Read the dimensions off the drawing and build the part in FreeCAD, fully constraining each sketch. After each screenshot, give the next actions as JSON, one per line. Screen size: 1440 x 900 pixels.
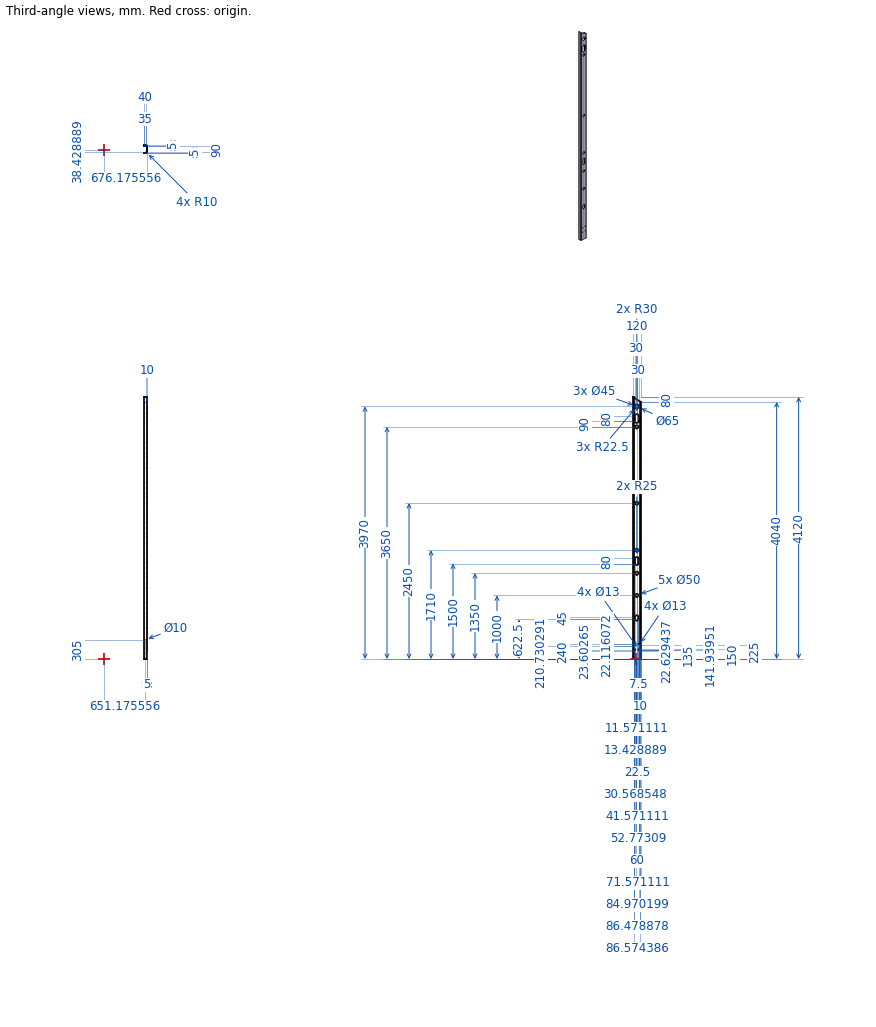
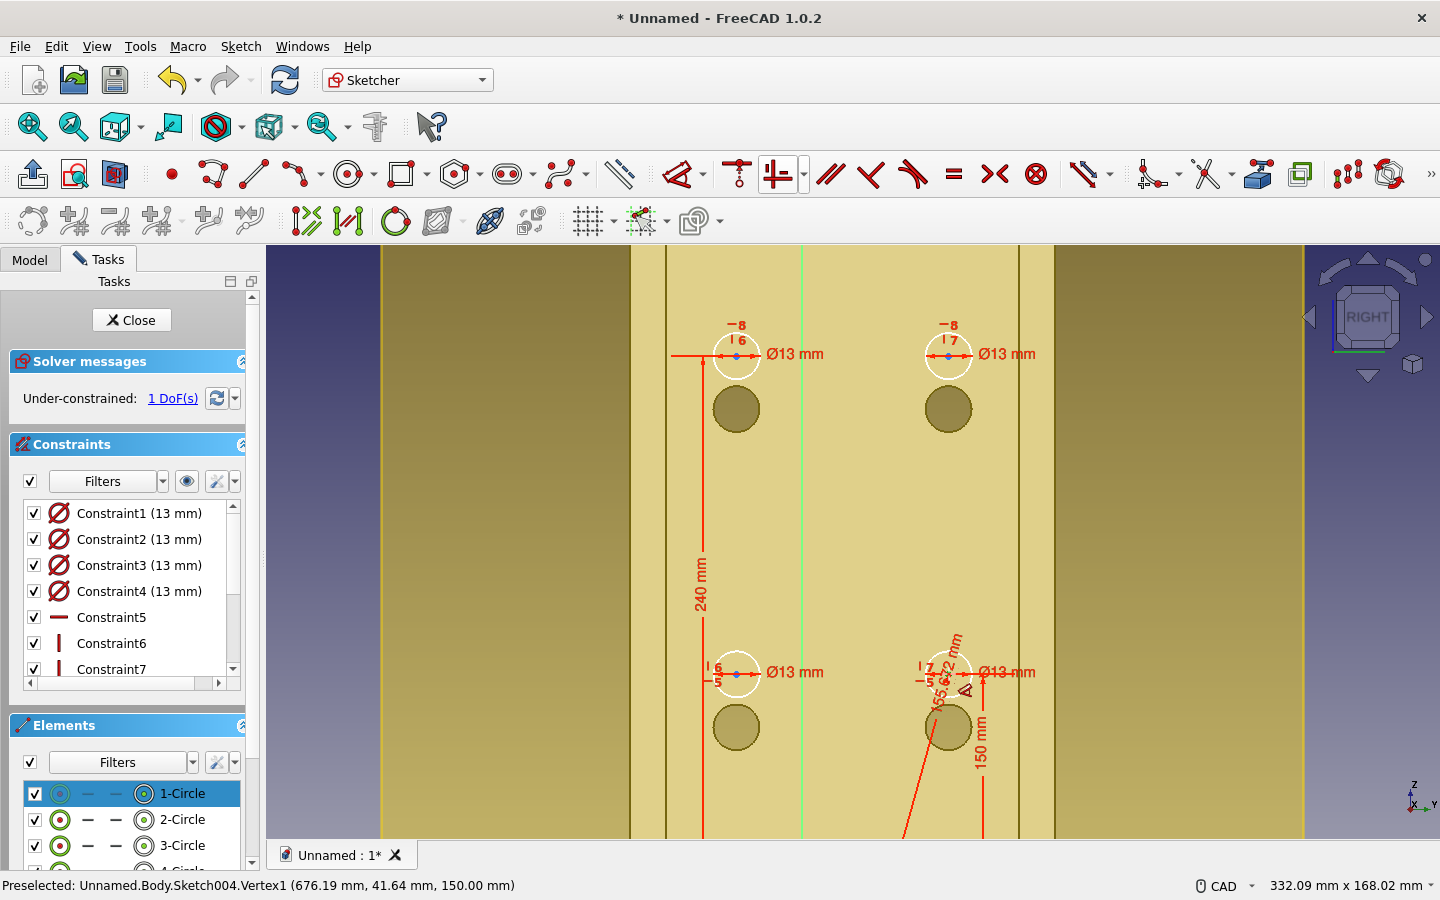
{"action": "left_click", "coordinate": [737, 674]}
{"action": "left_click", "coordinate": [843, 640]}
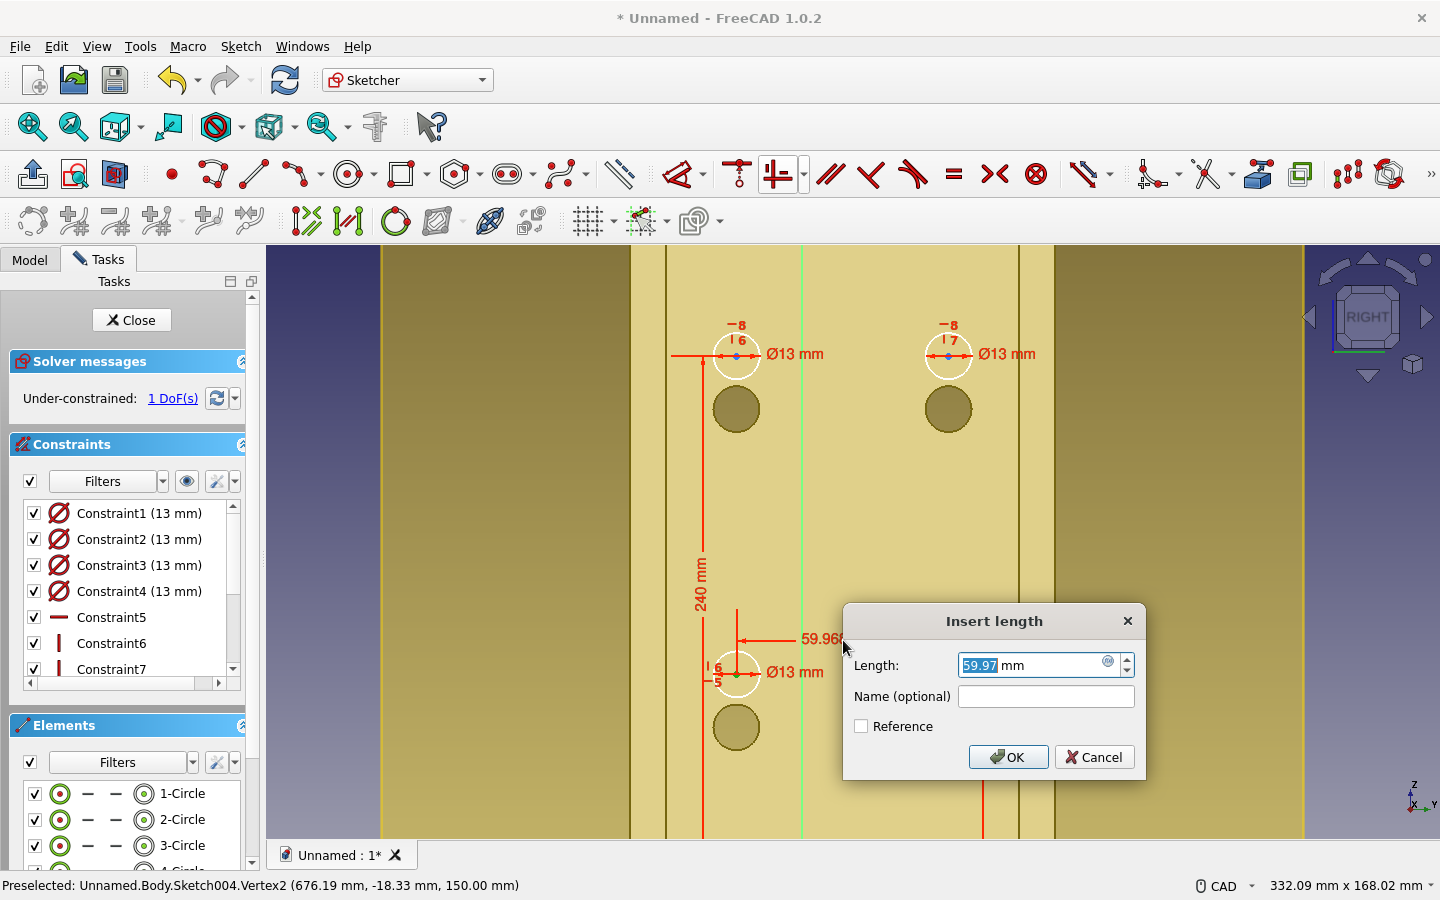
{"action": "type", "text": "60"}
{"action": "key", "text": "Return"}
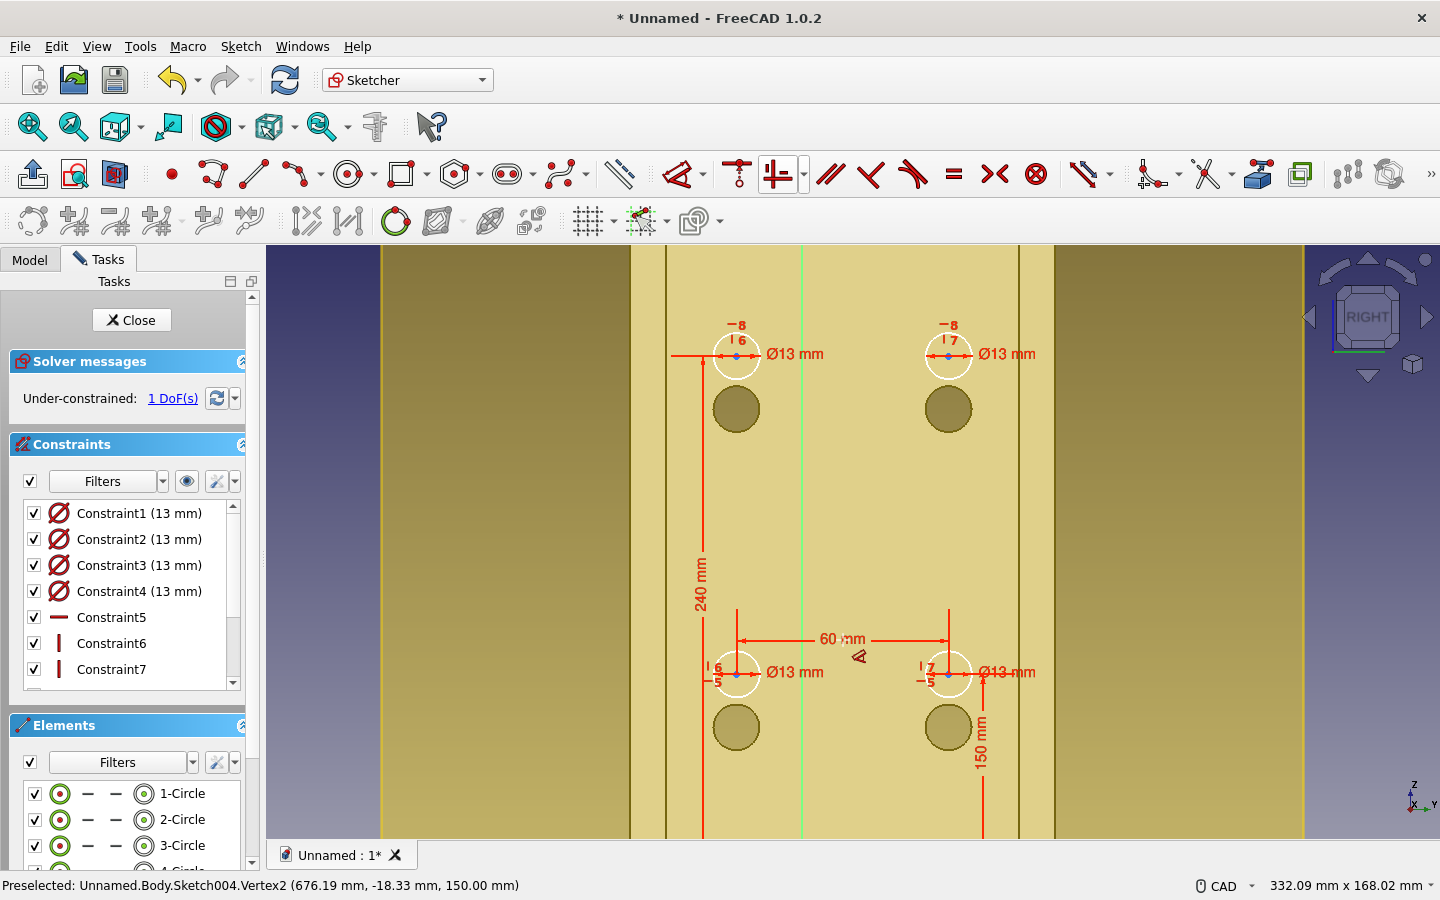
{"action": "left_click", "coordinate": [949, 674]}
{"action": "left_click", "coordinate": [927, 640]}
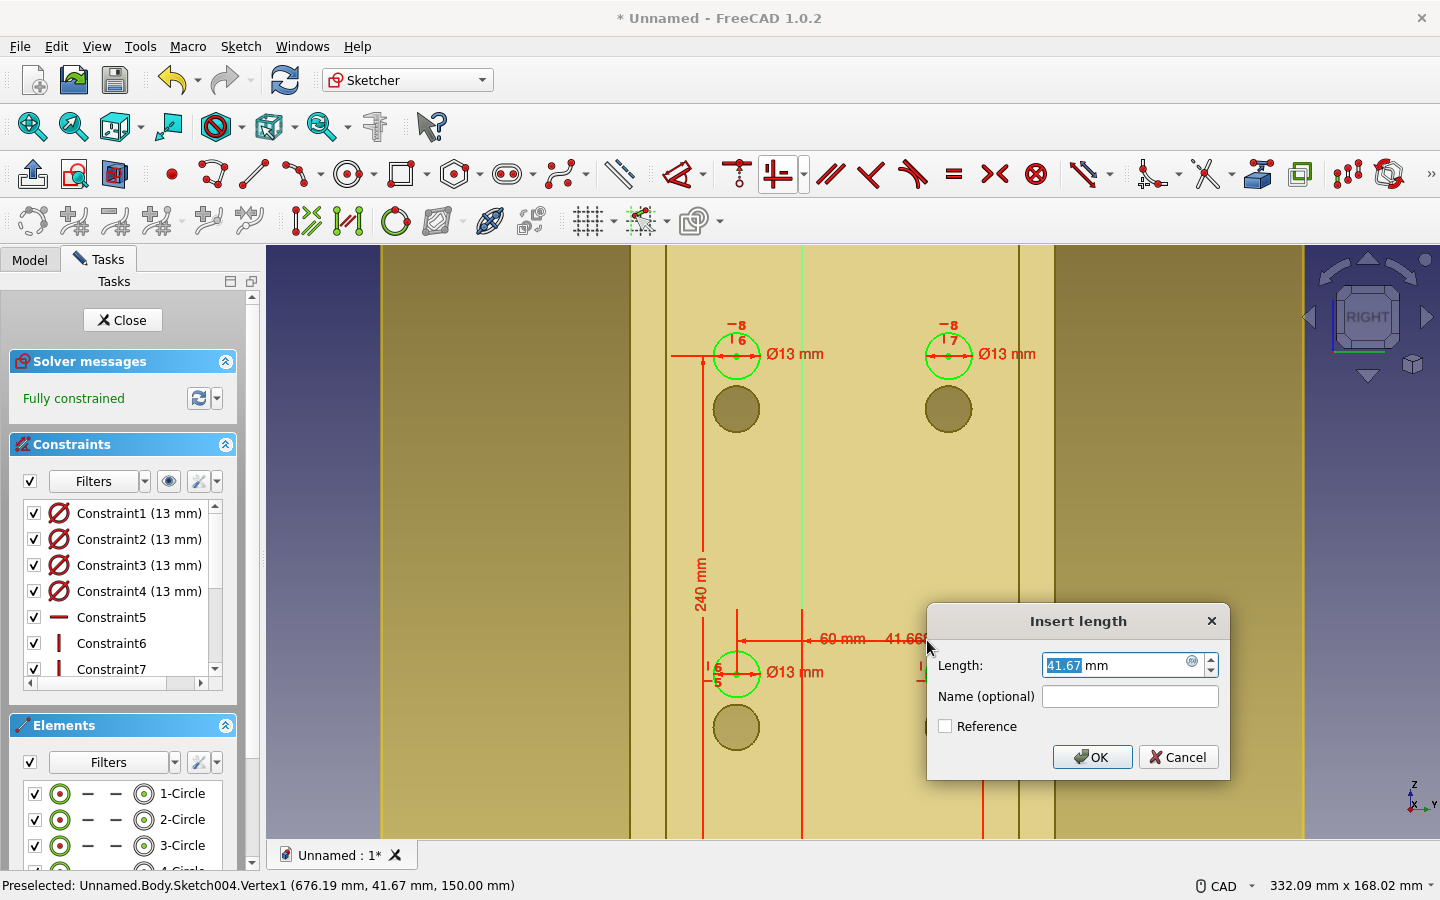
{"action": "type", "text": "41.571111"}
{"action": "key", "text": "Return"}
{"action": "key", "text": "Escape"}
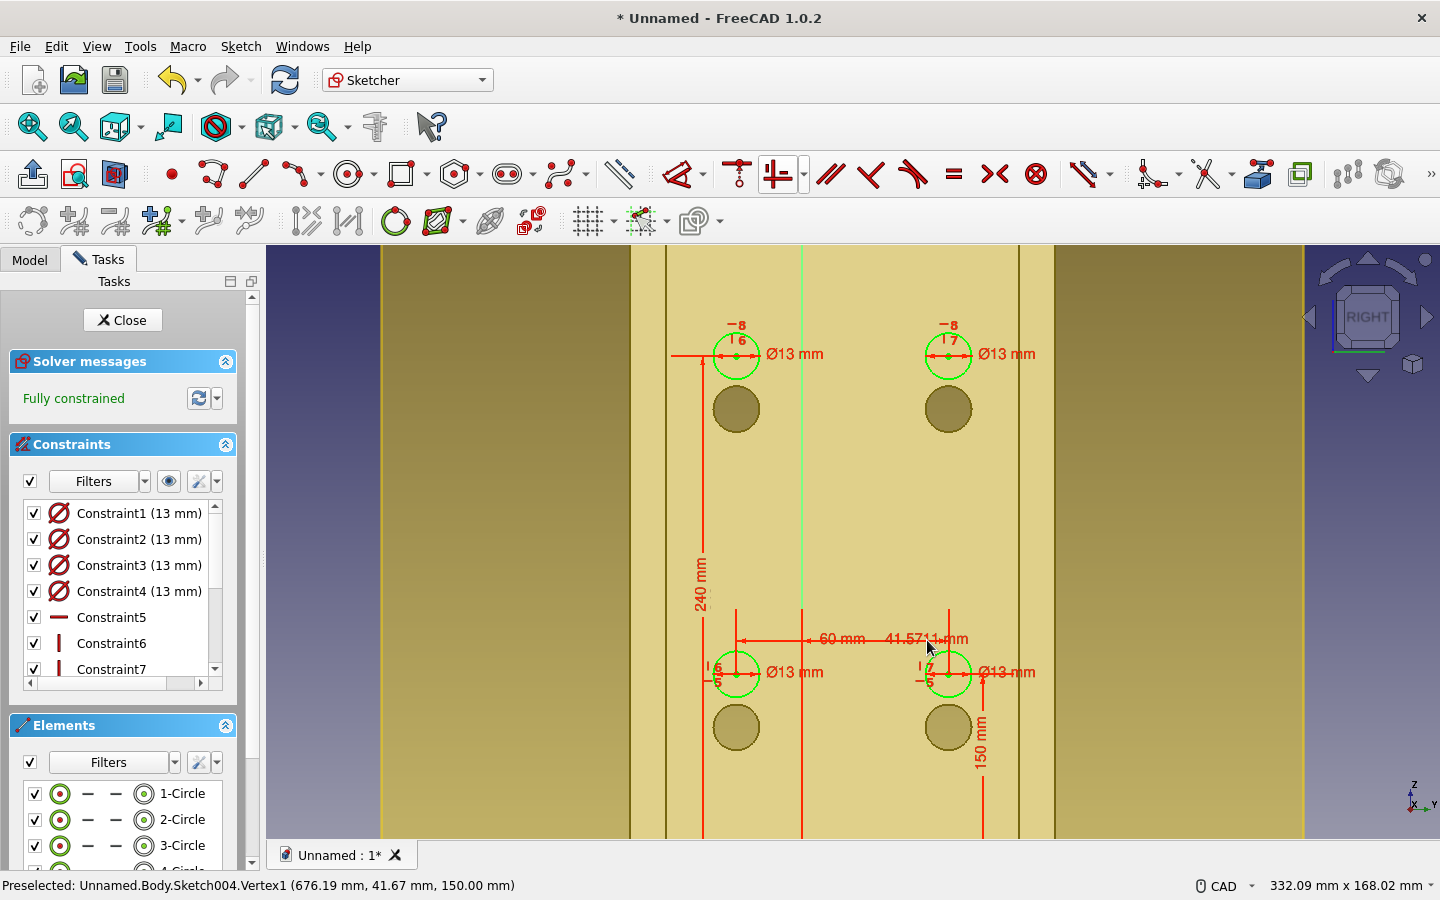
{"action": "left_click", "coordinate": [123, 320]}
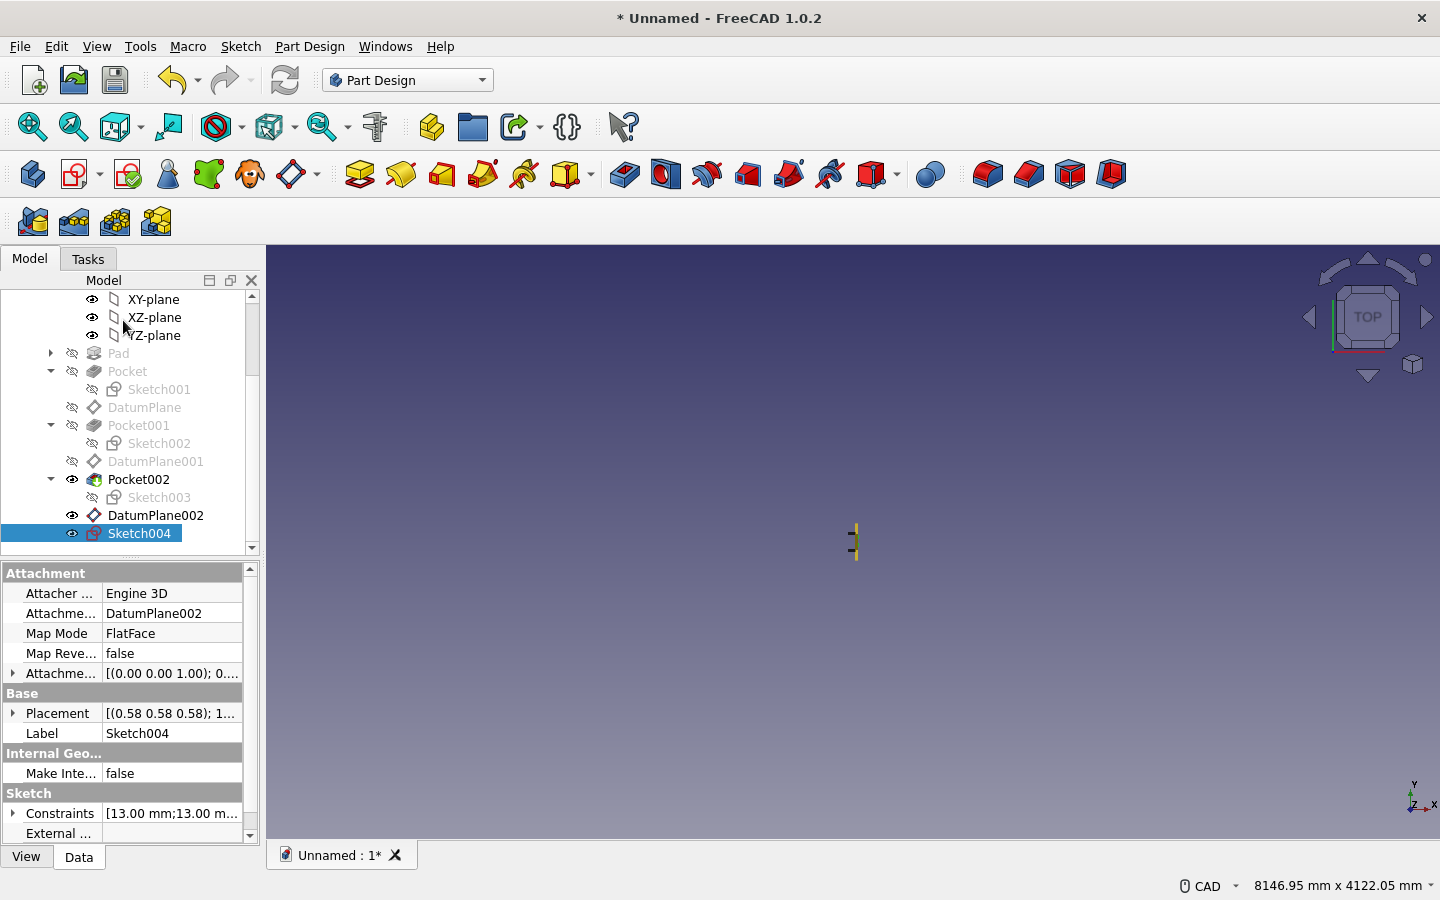
{"action": "left_click", "coordinate": [625, 174]}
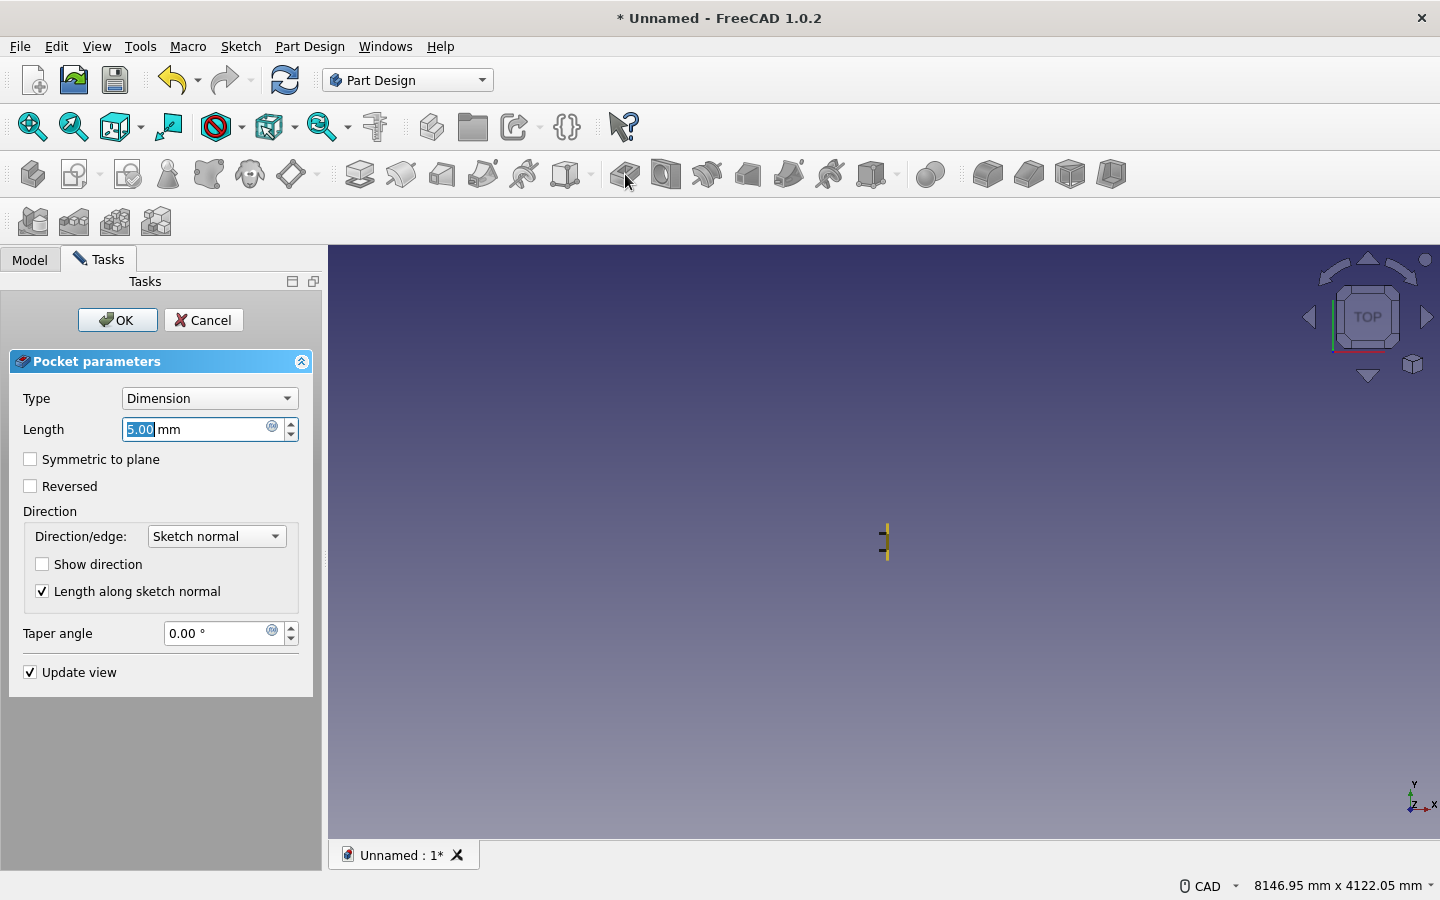
{"action": "type", "text": "10"}
{"action": "key", "text": "Tab"}